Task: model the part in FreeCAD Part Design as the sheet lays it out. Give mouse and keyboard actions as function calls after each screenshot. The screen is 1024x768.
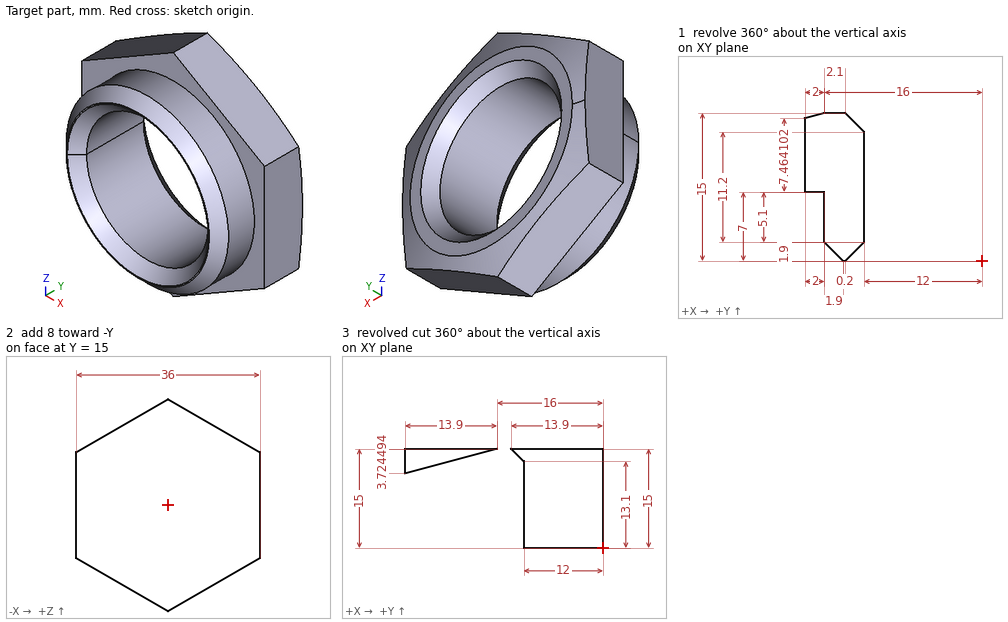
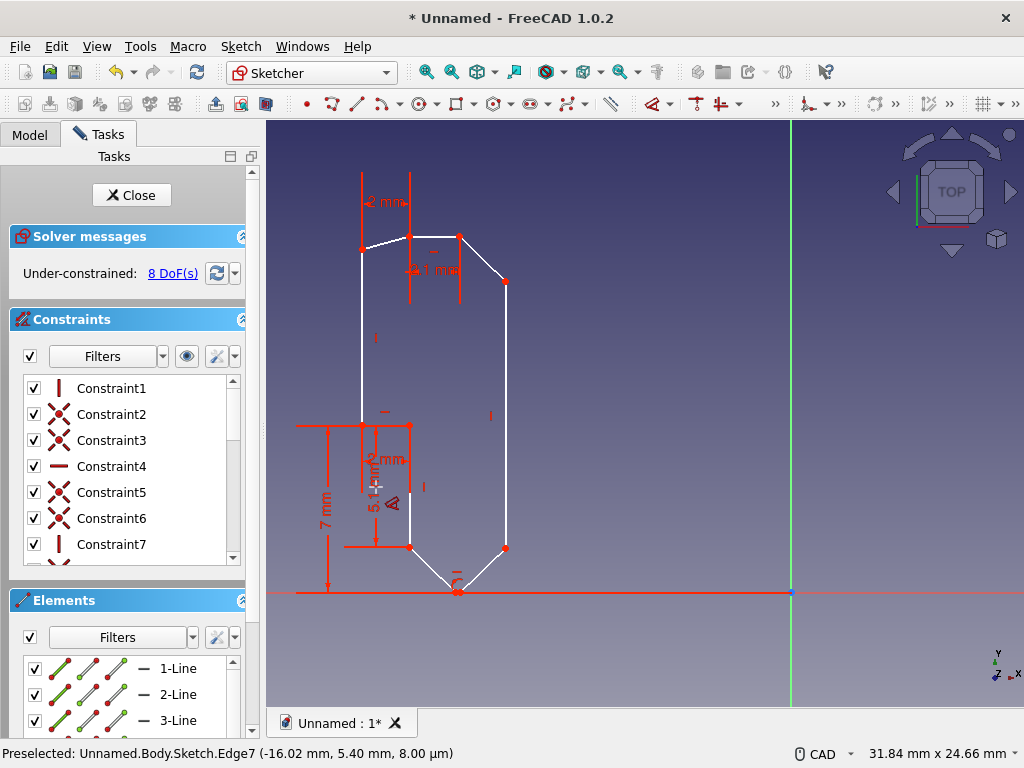
scroll(458, 593, up, 11)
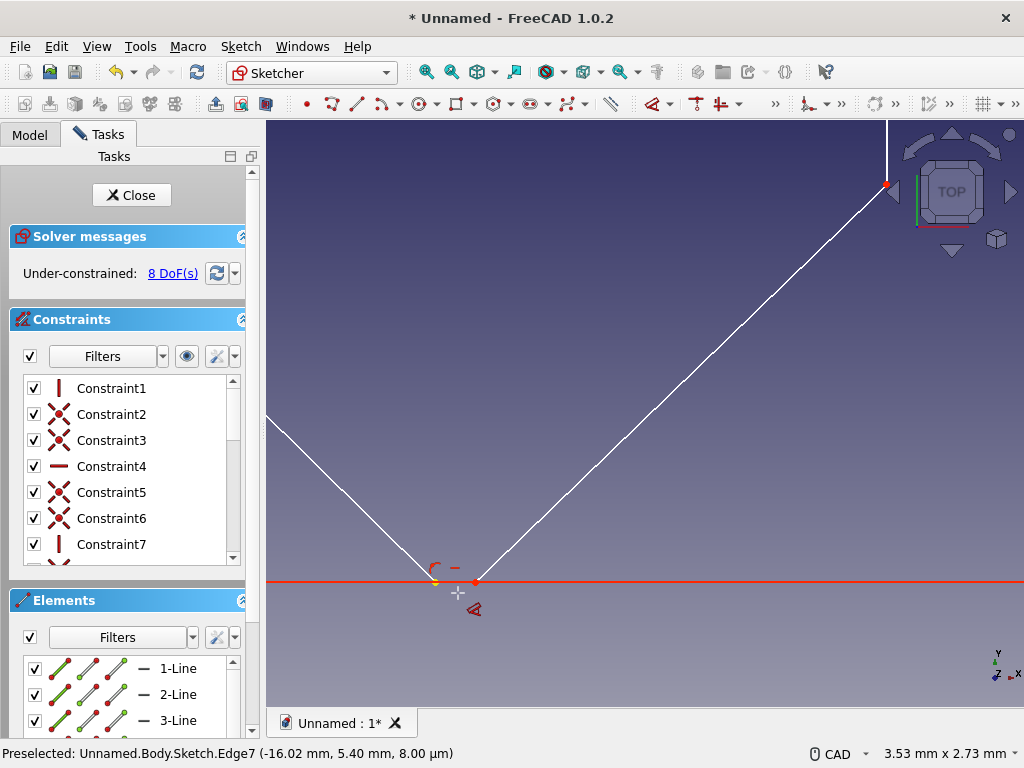
click(456, 582)
click(456, 616)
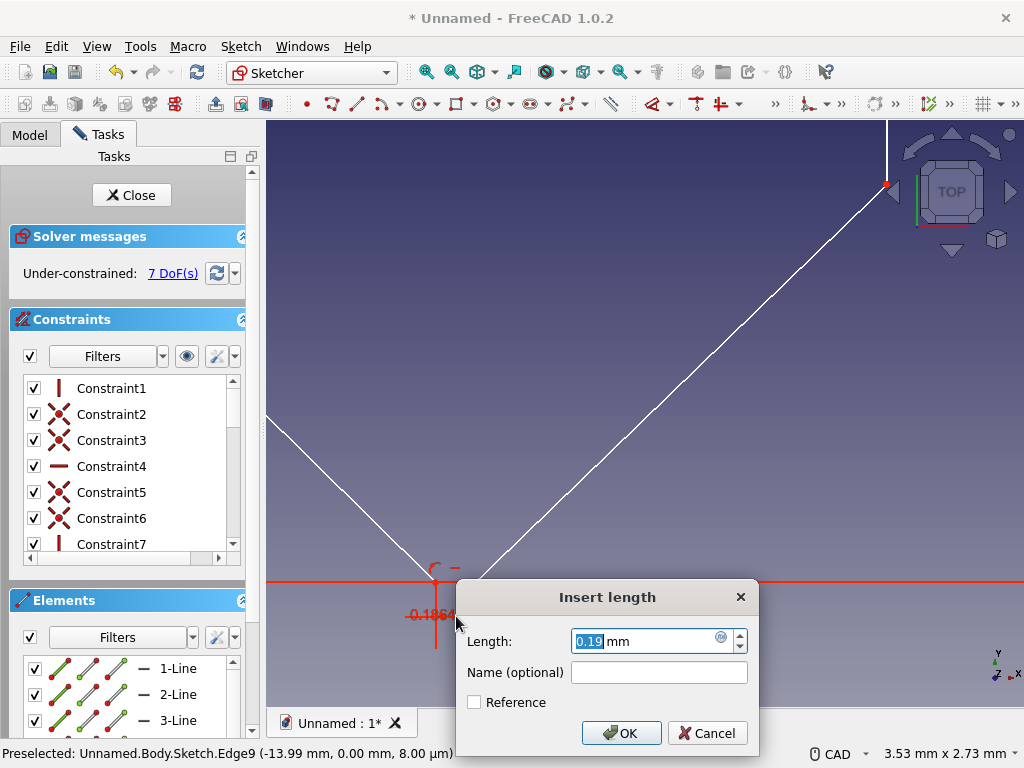
text(0.2)
key(Return)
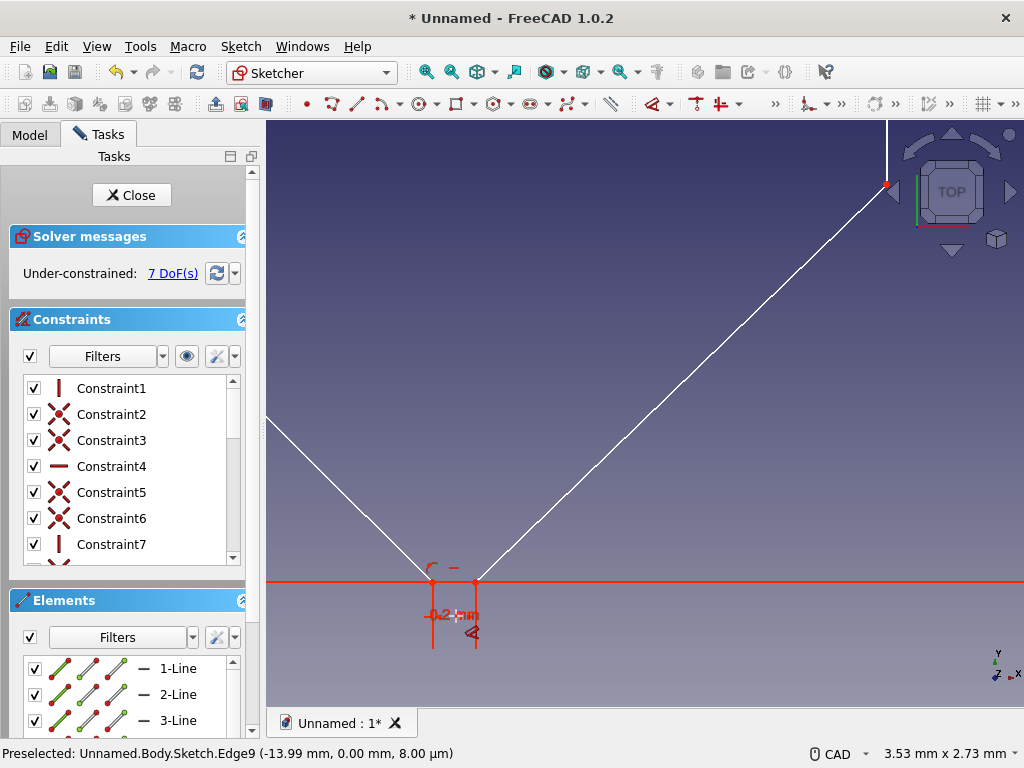
scroll(458, 593, down, 11)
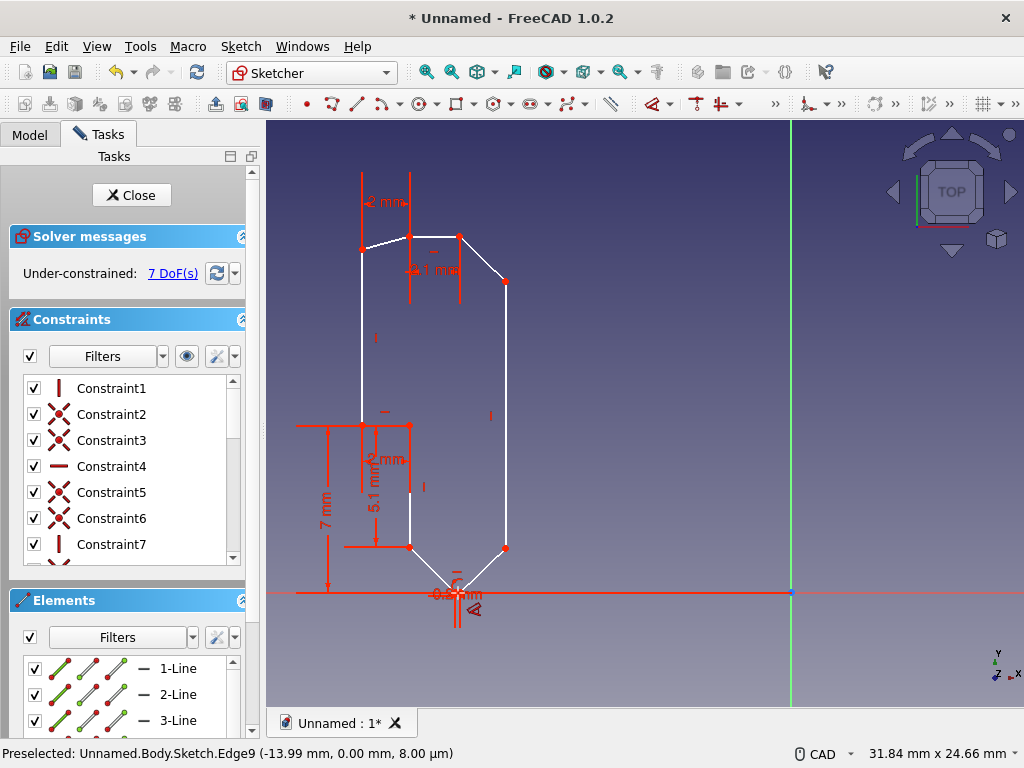
click(506, 549)
click(648, 627)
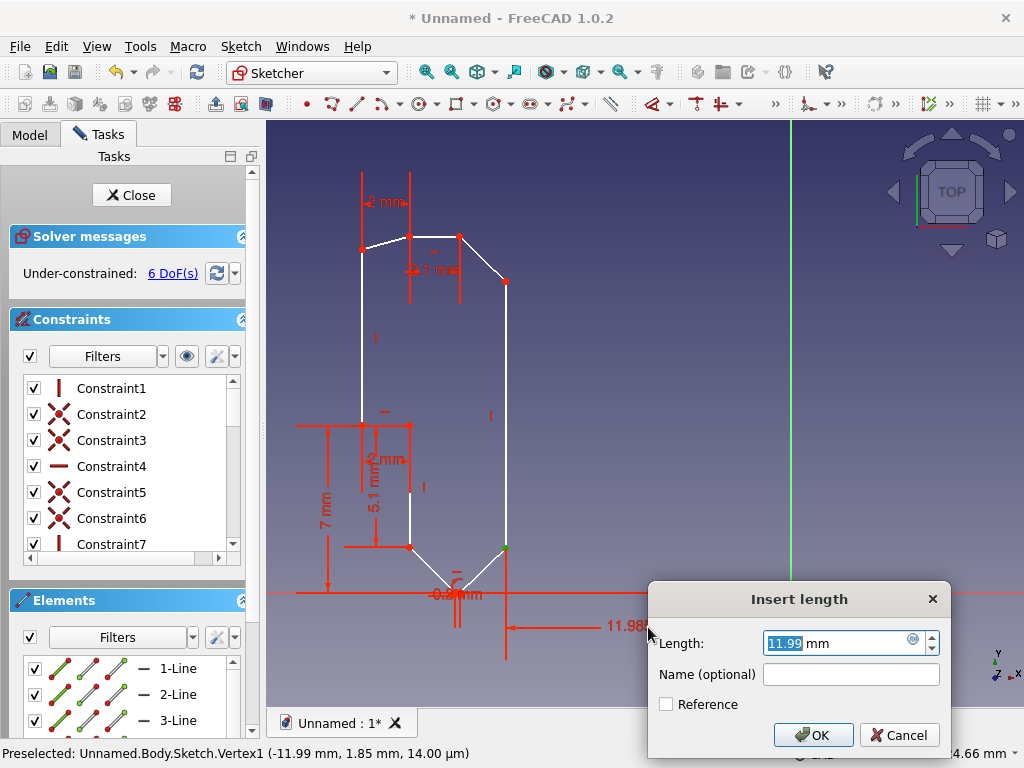
text(12)
key(Return)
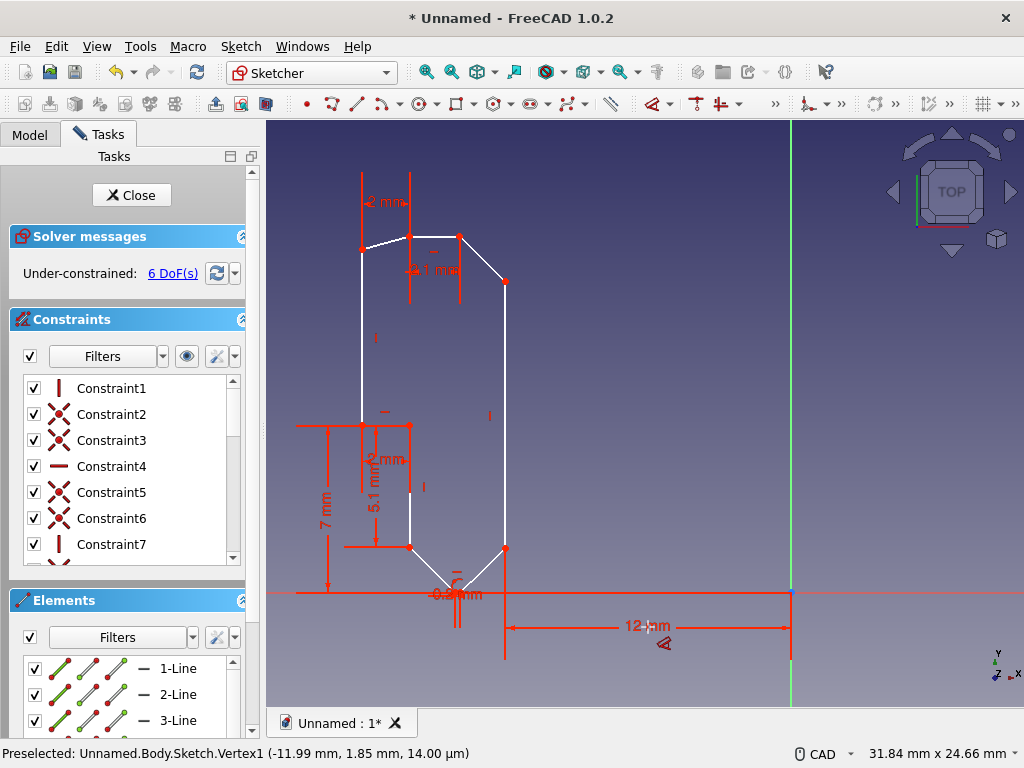
click(460, 237)
click(825, 415)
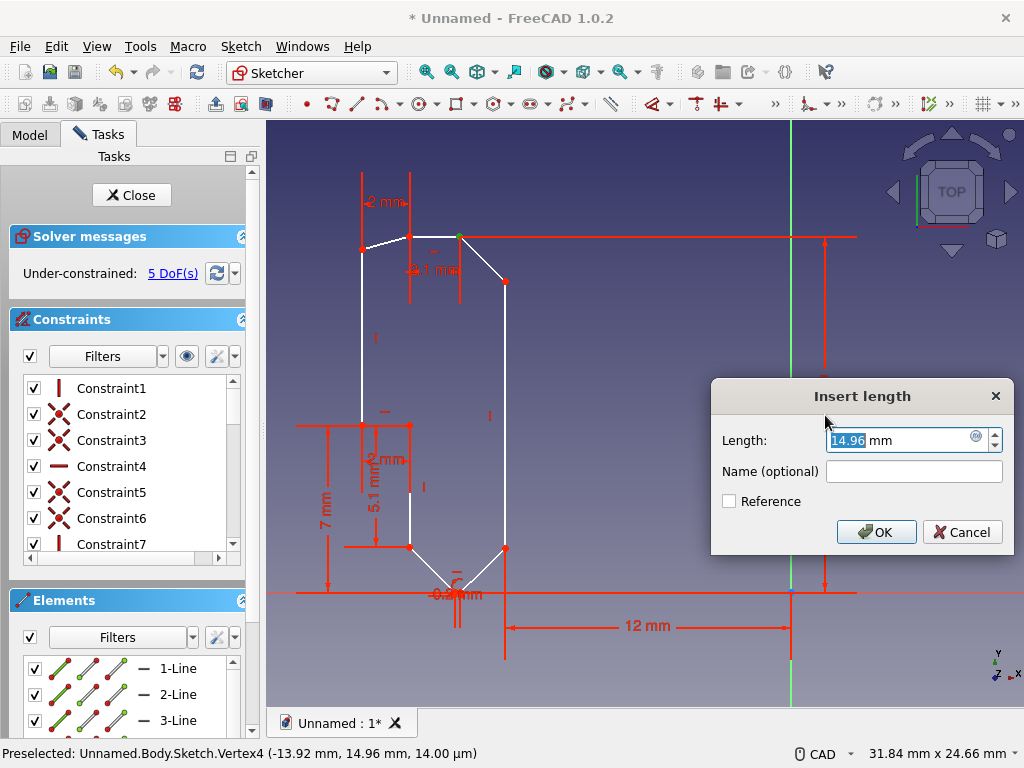
text(15)
key(Return)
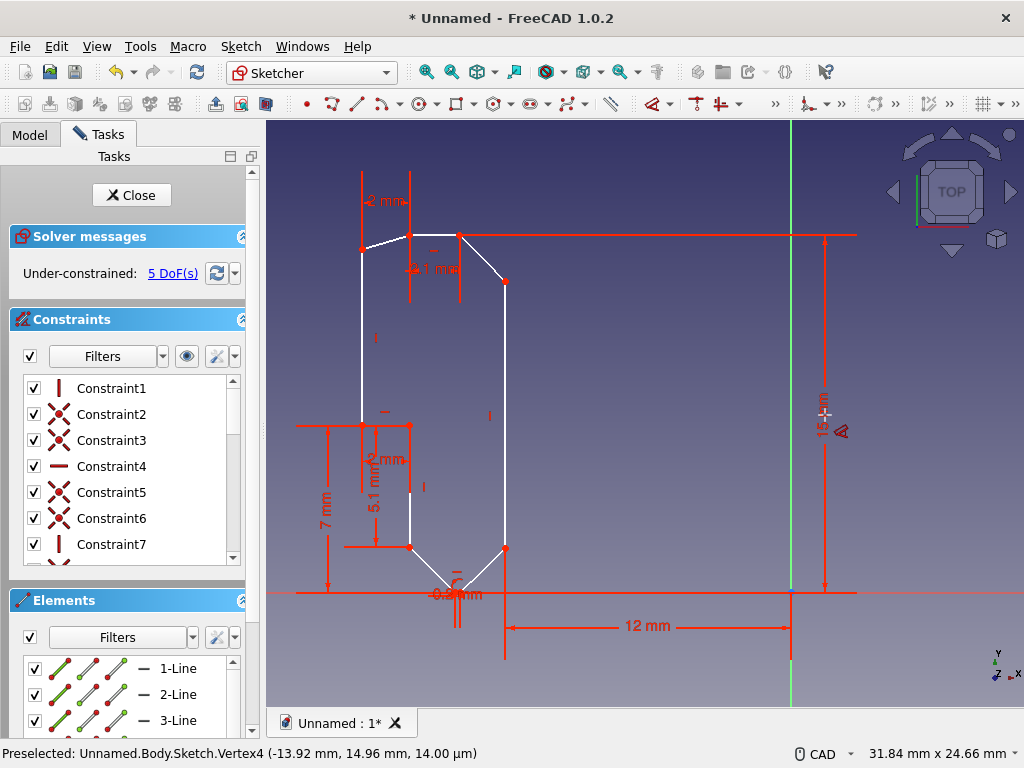
click(410, 235)
click(513, 627)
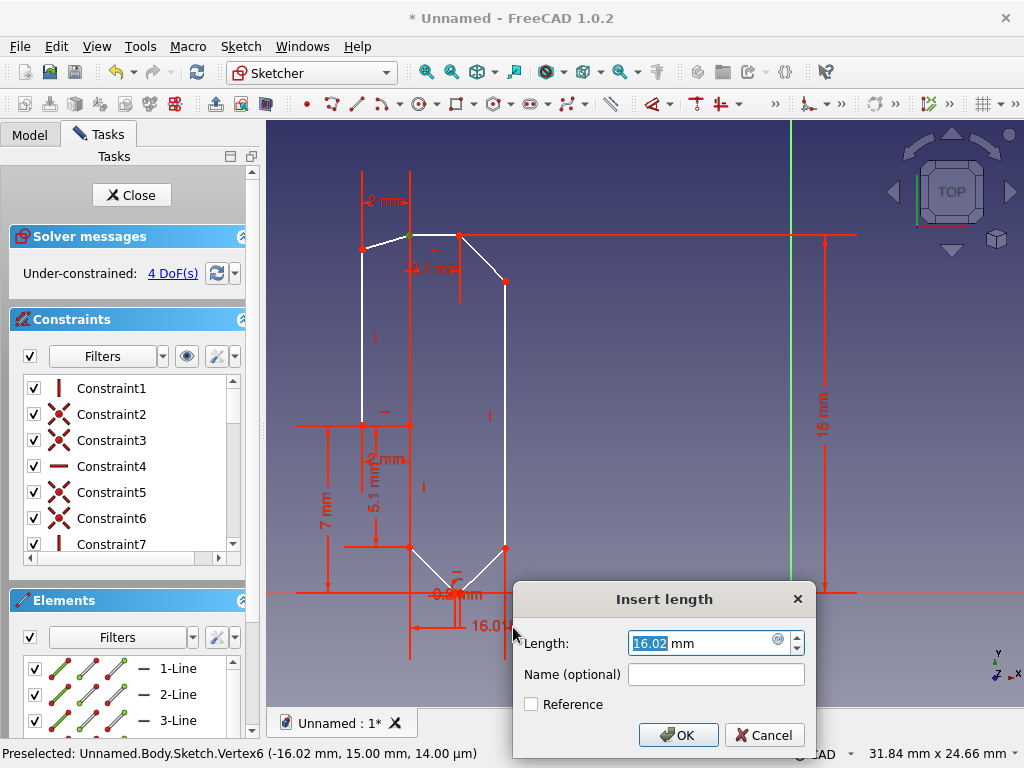
text(16)
key(Return)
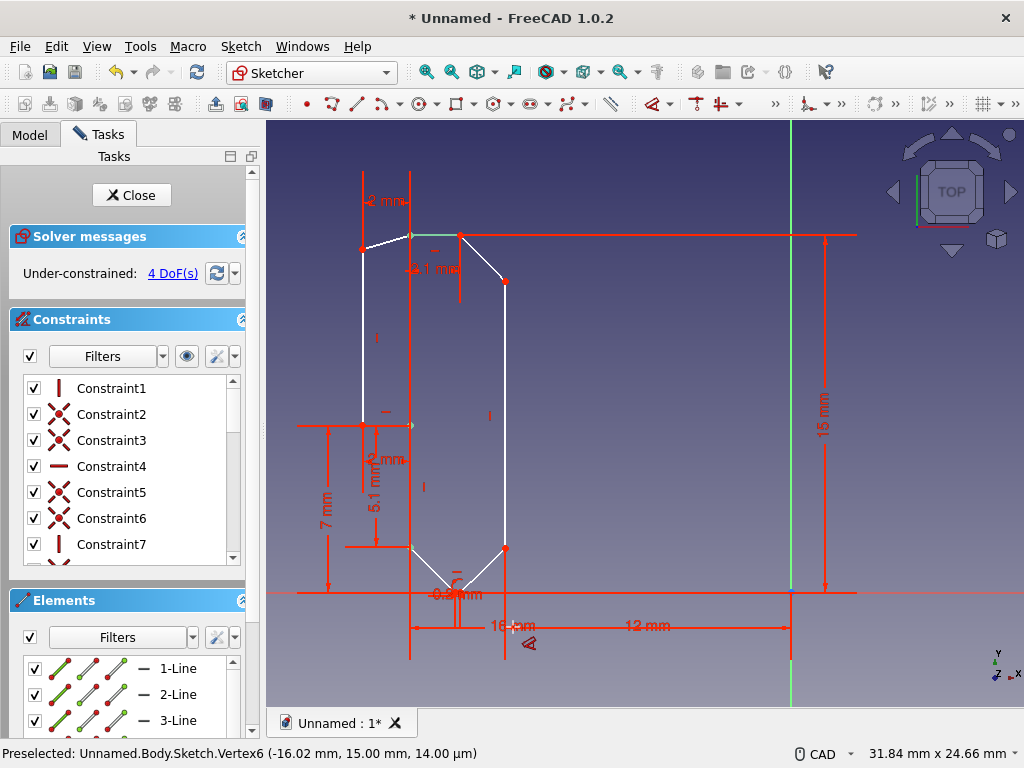
click(505, 468)
click(471, 415)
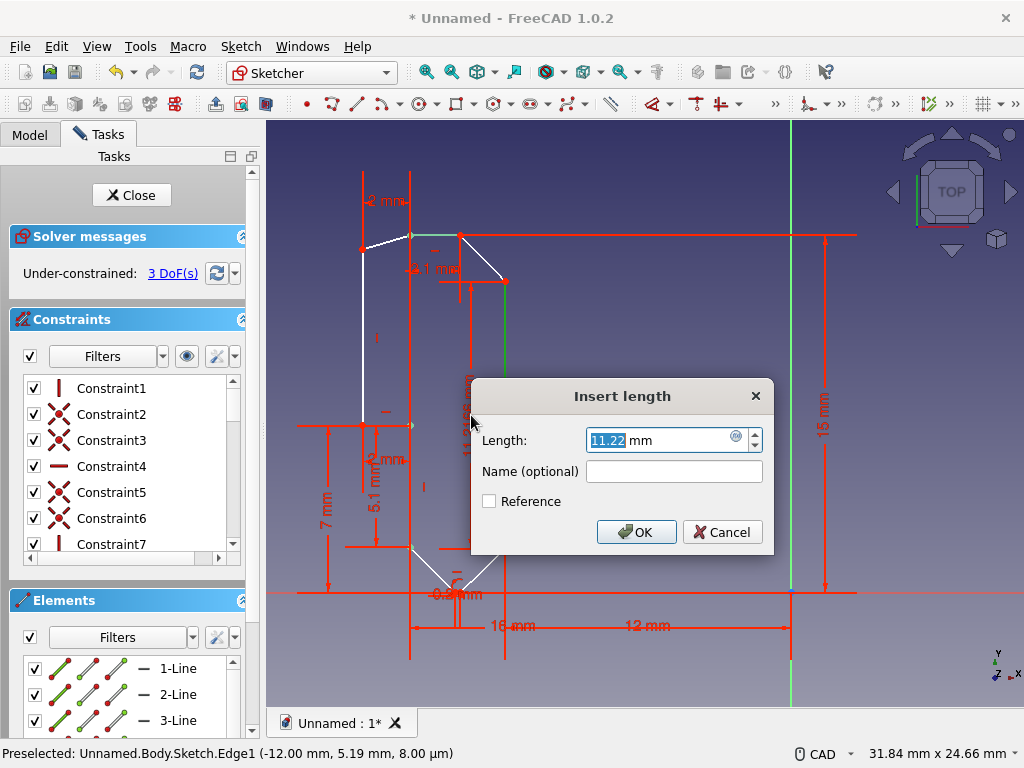
text(11.2)
key(Return)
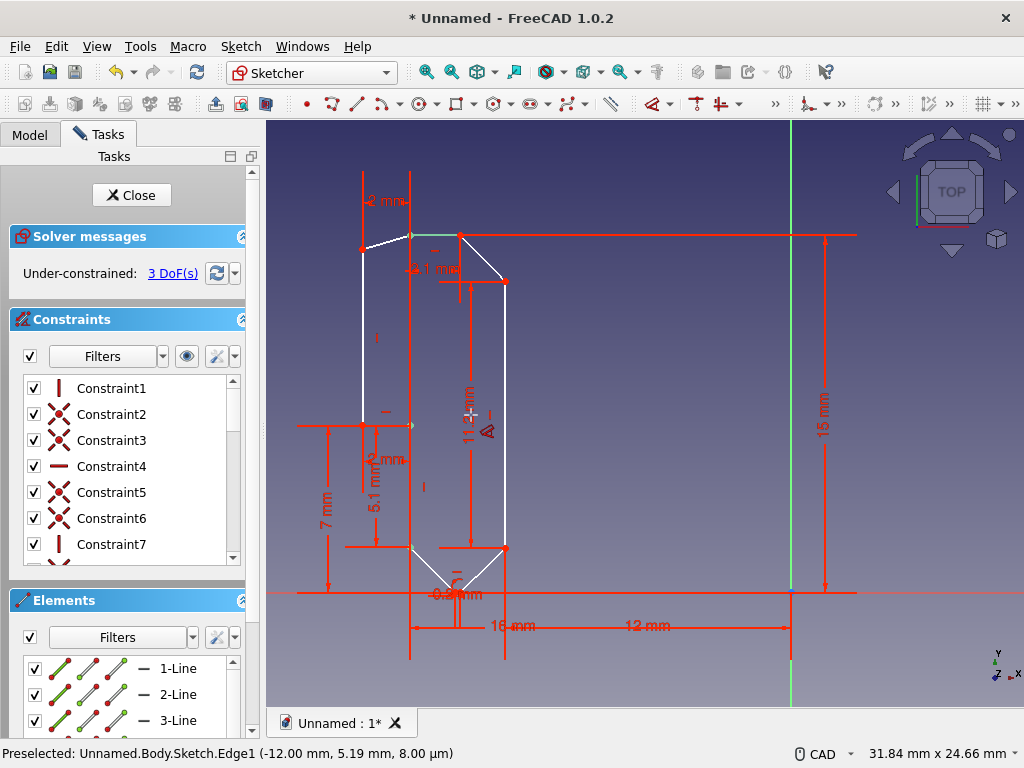
click(505, 548)
click(825, 570)